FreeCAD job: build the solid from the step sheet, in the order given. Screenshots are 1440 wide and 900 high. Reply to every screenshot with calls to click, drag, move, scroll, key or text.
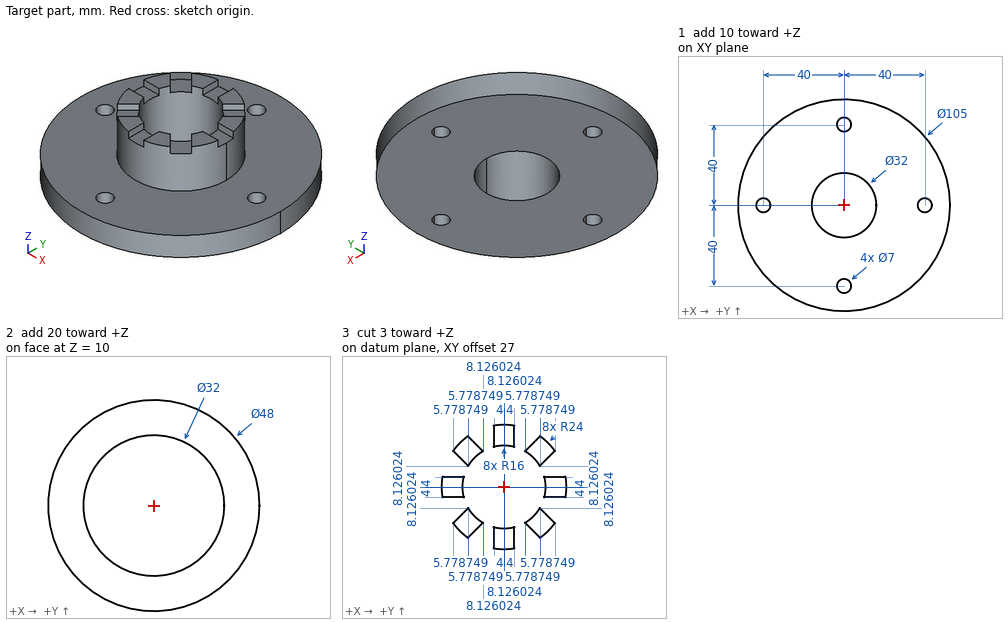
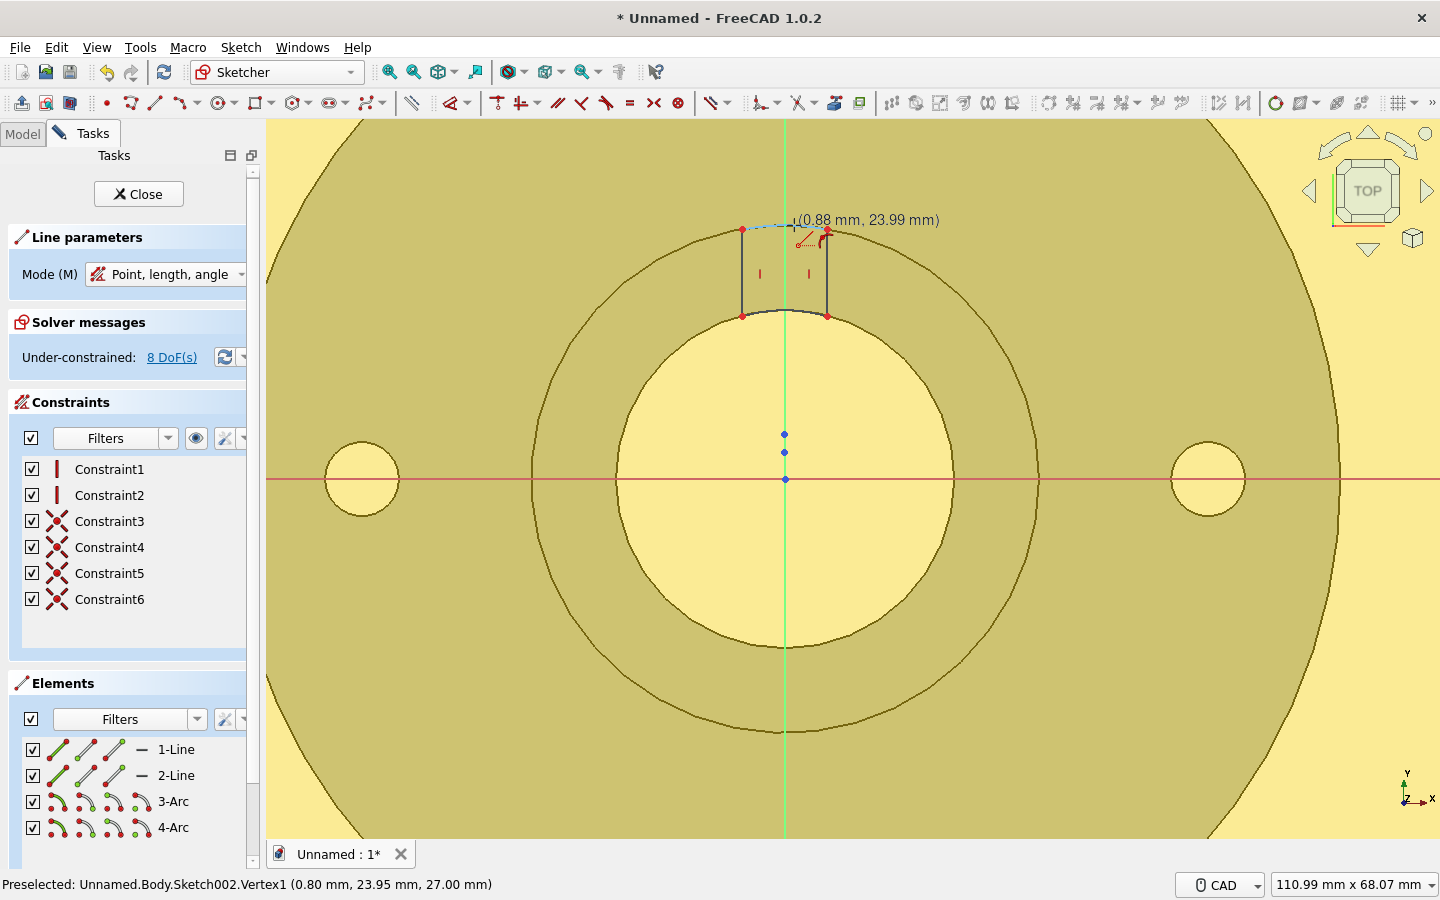
click(932, 272)
click(871, 333)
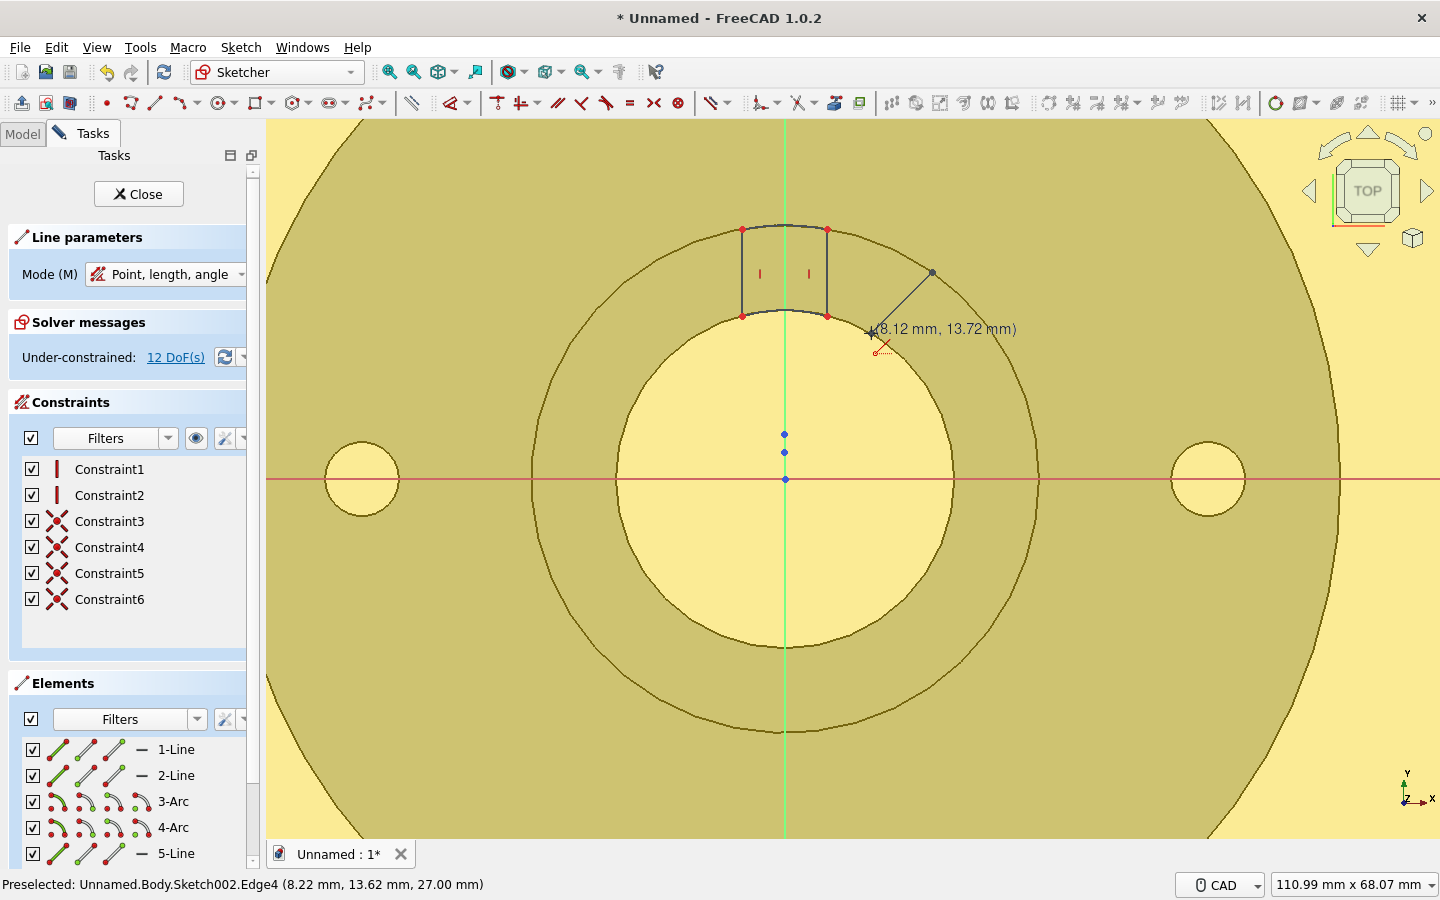
click(931, 393)
click(992, 332)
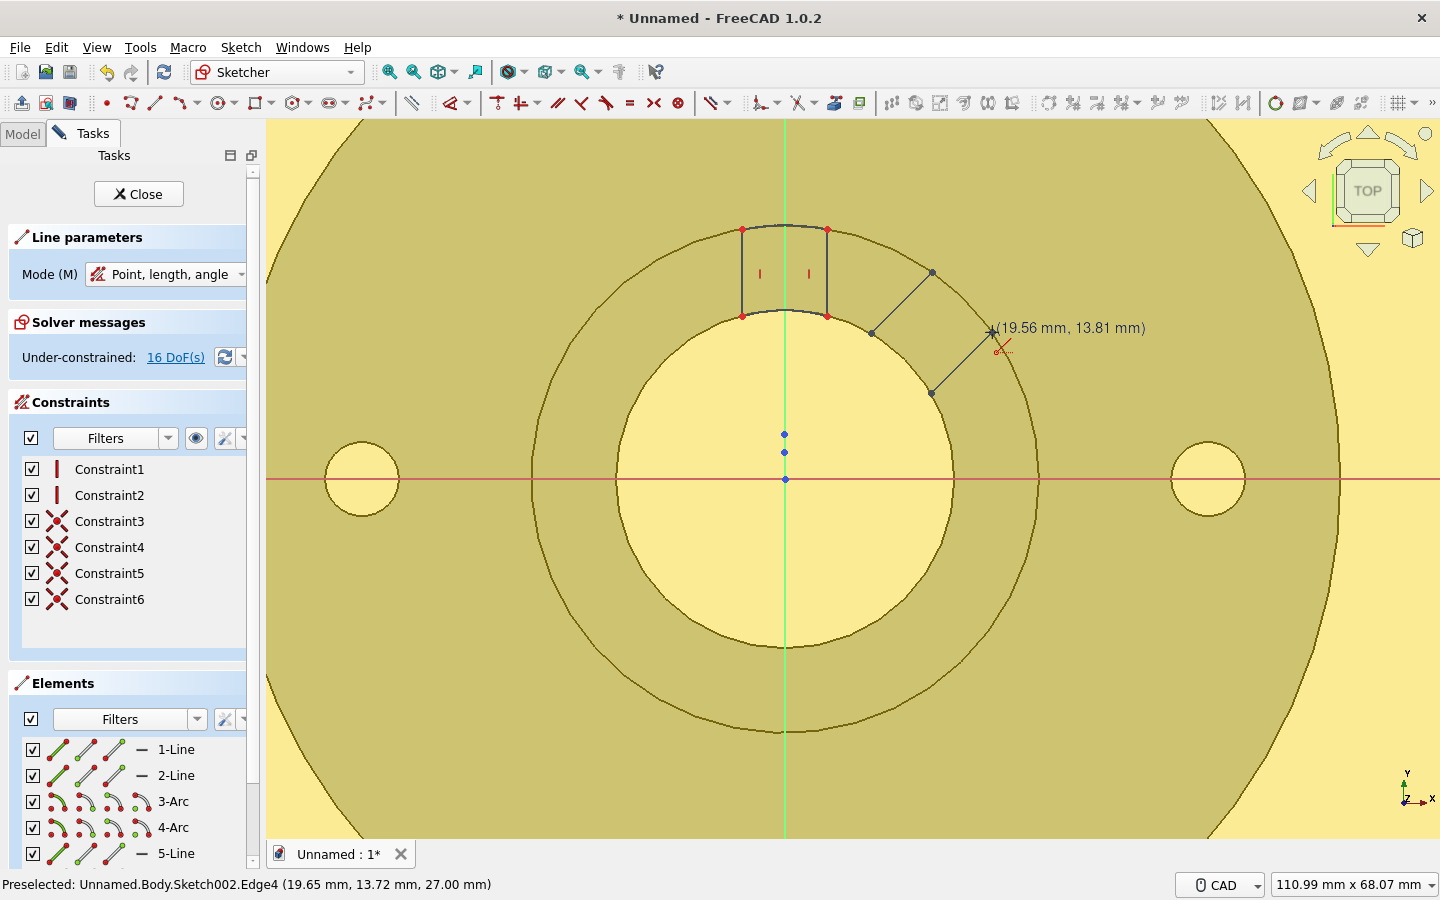
click(180, 104)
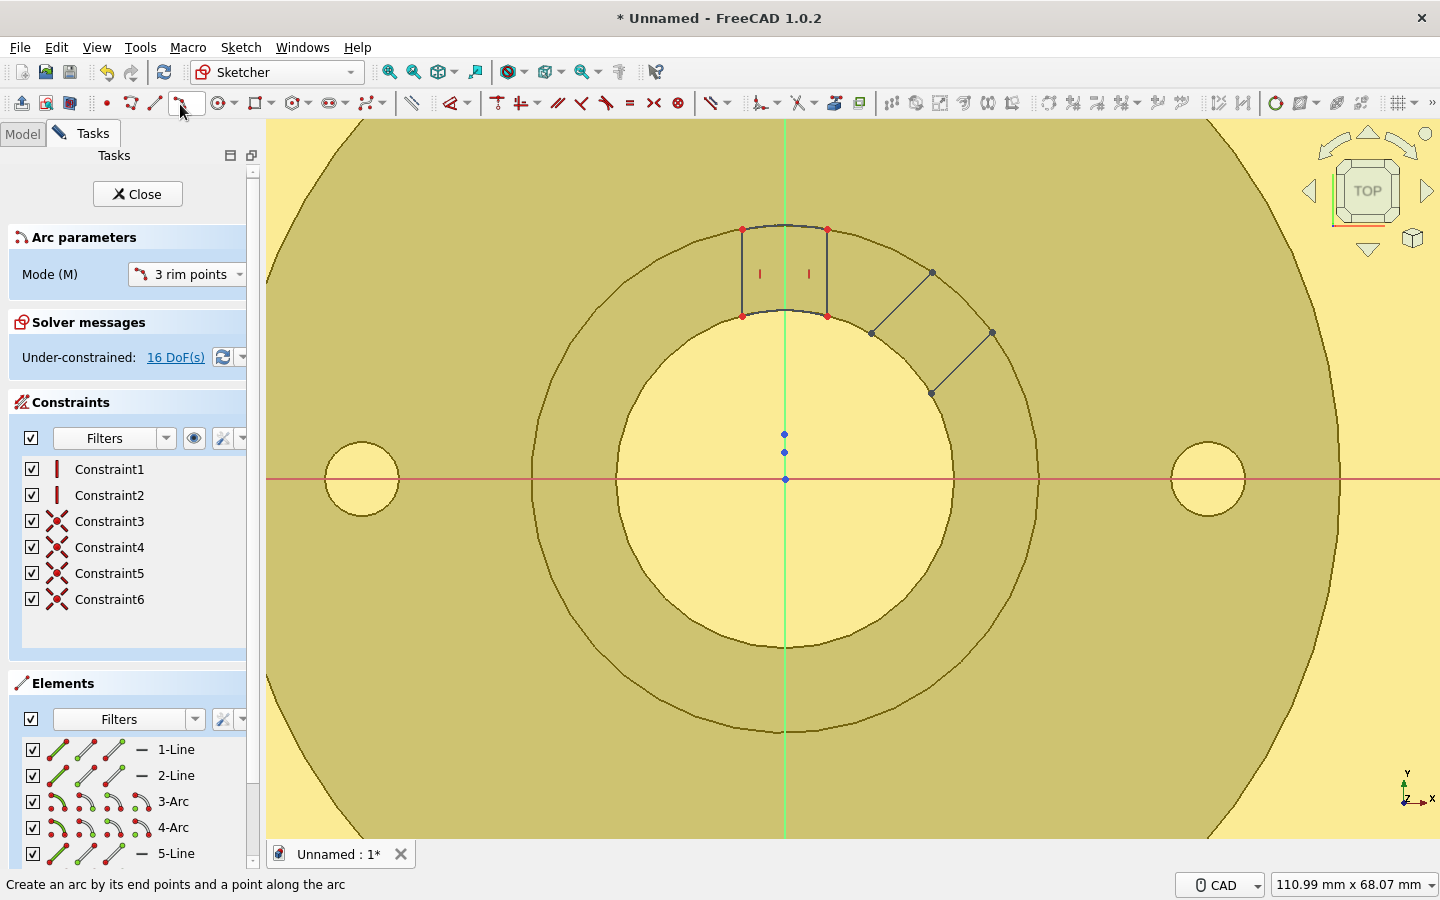
click(871, 334)
click(931, 394)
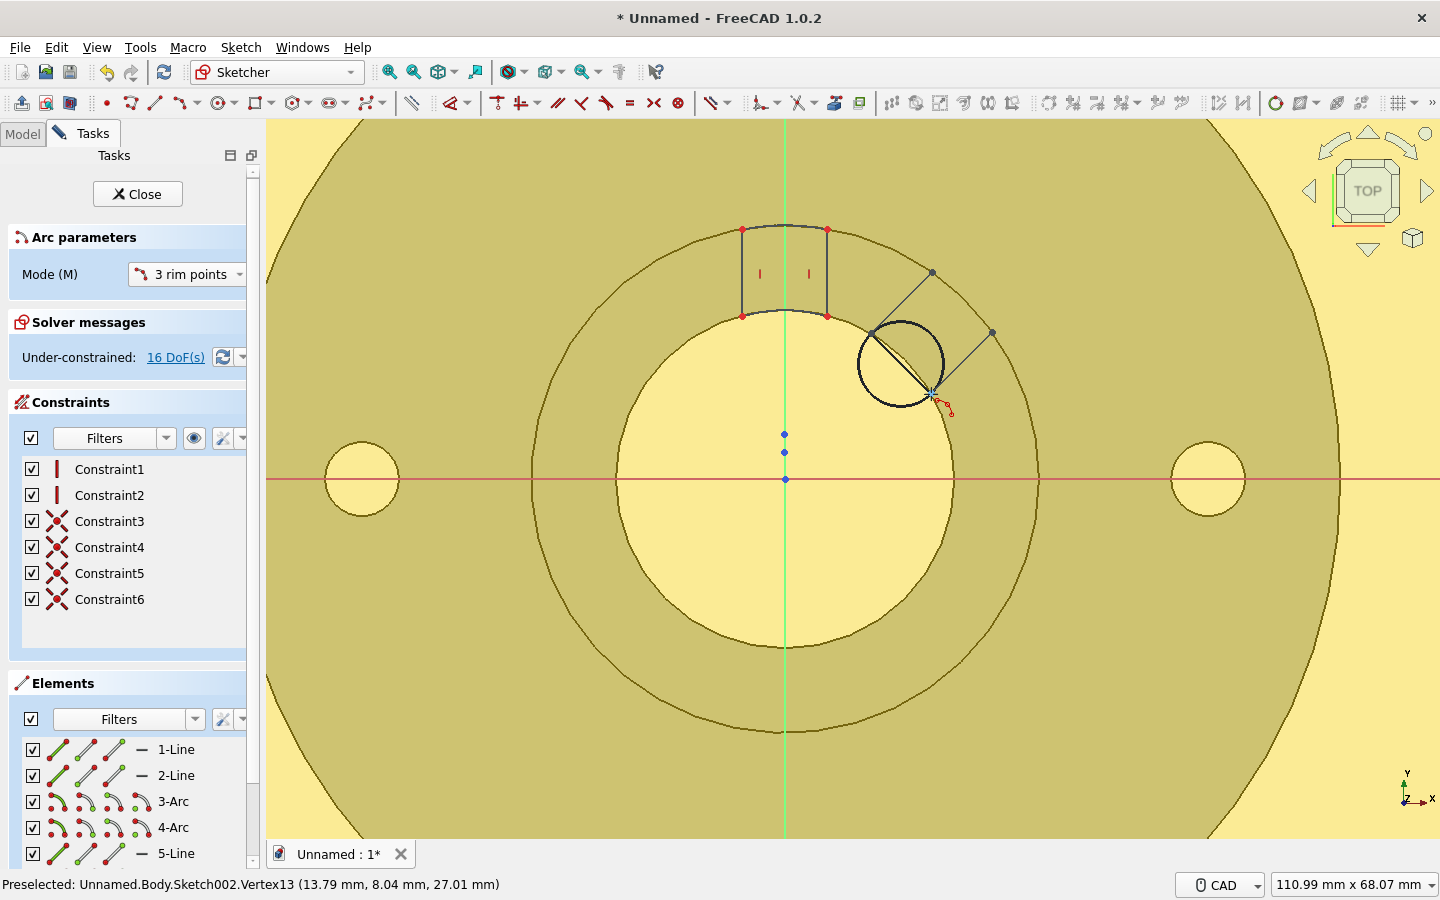
scroll(905, 359, up, 6)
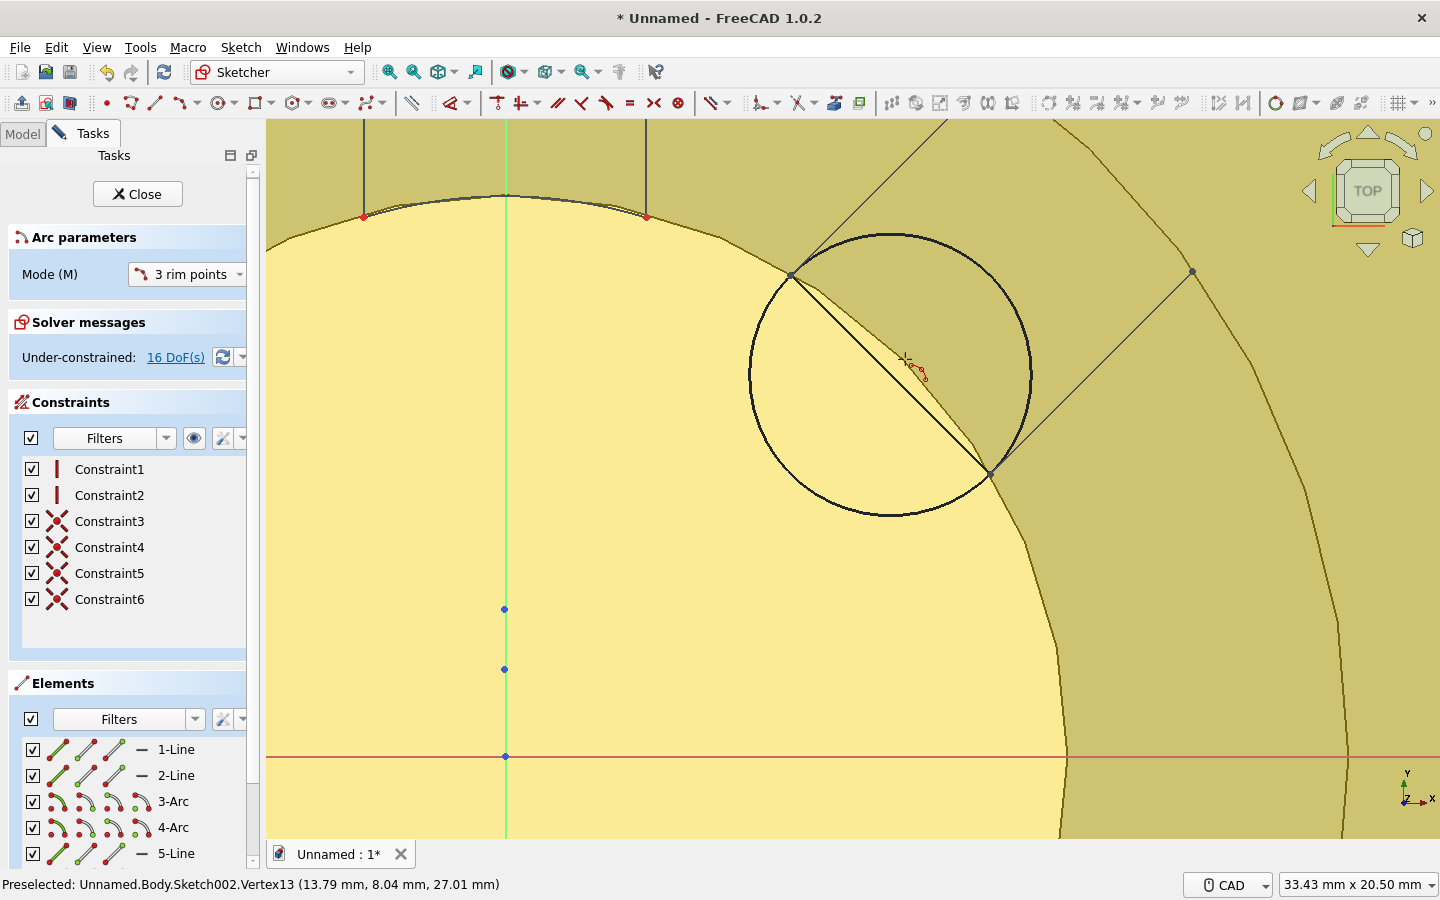
click(903, 360)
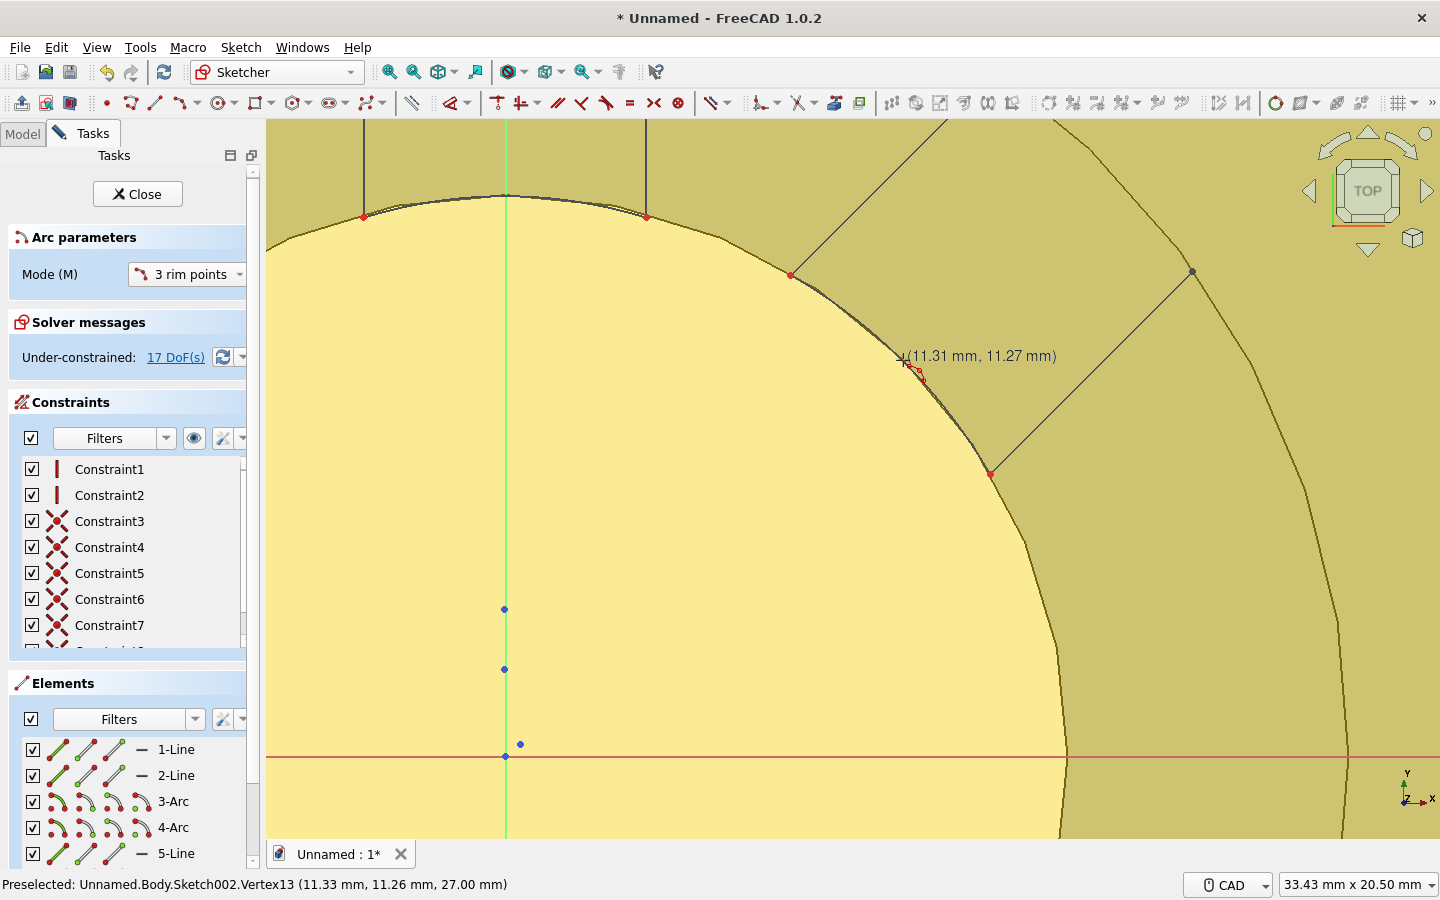
click(1193, 272)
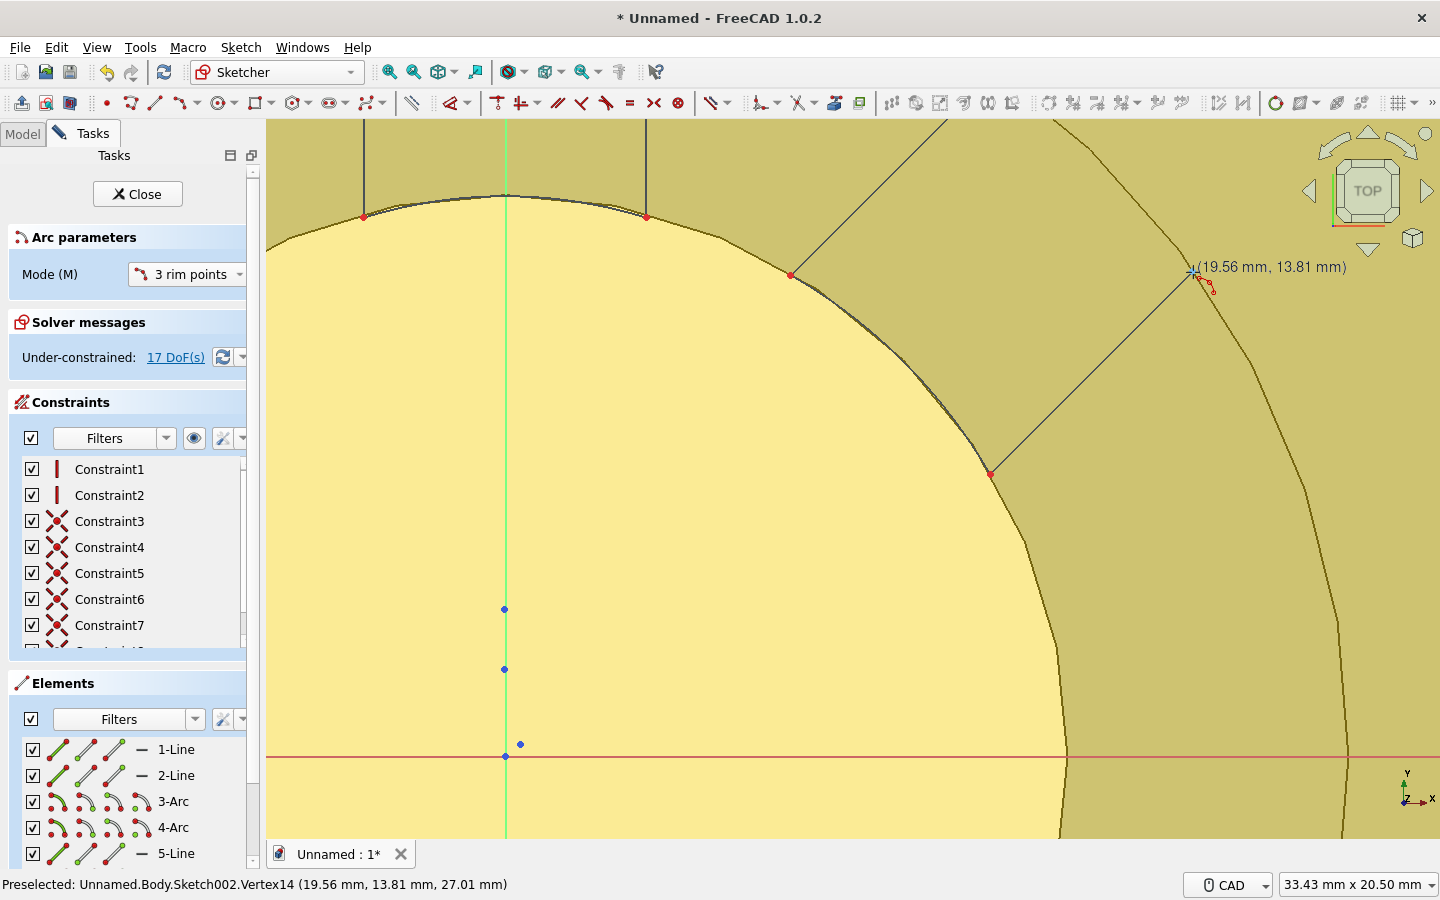
scroll(905, 359, down, 6)